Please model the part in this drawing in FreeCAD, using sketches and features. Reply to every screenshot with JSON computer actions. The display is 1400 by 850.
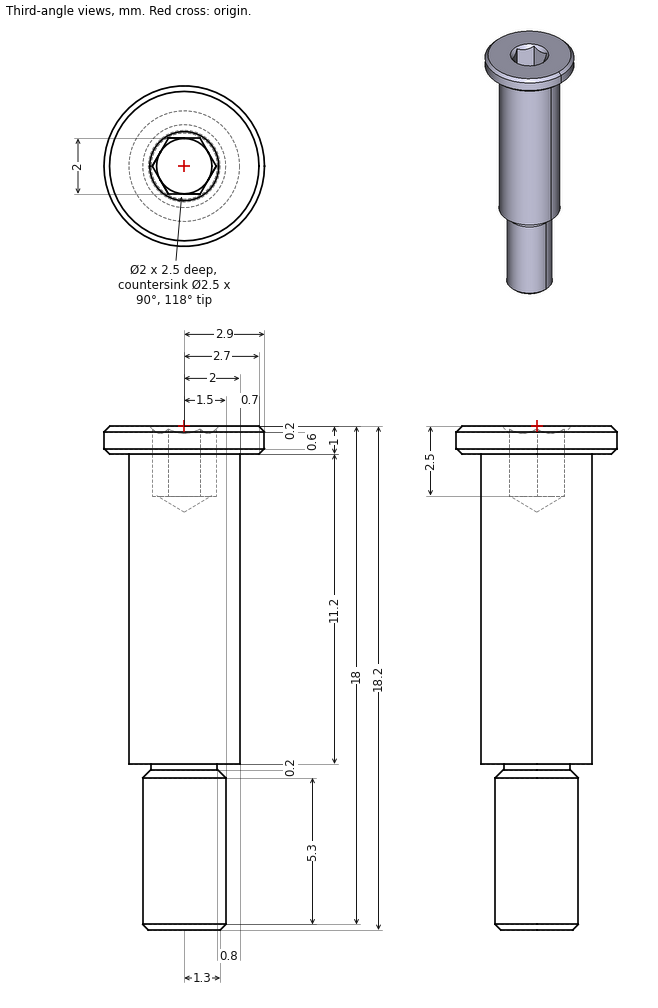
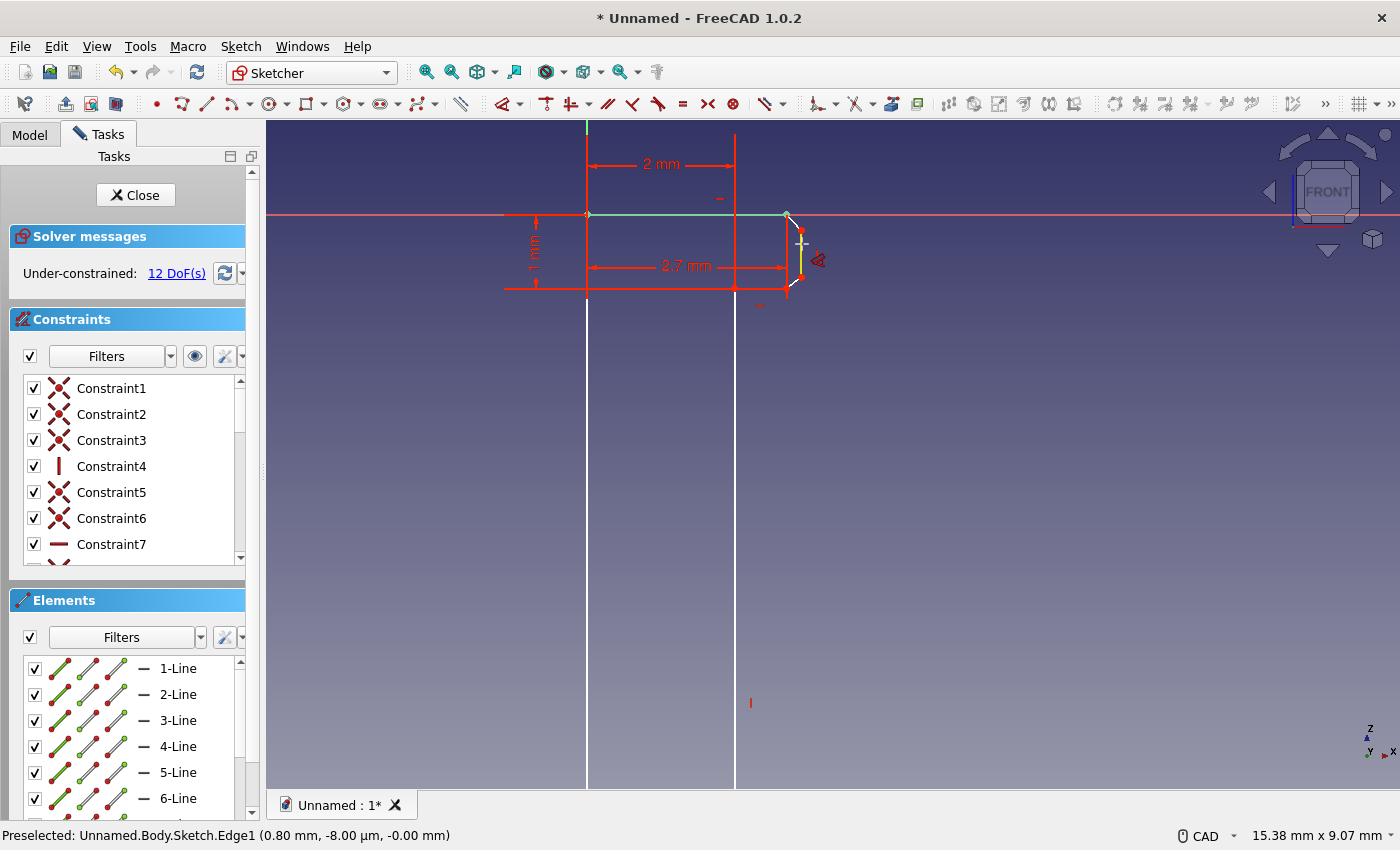
{"action": "left_click", "coordinate": [801, 244]}
{"action": "left_click", "coordinate": [835, 254]}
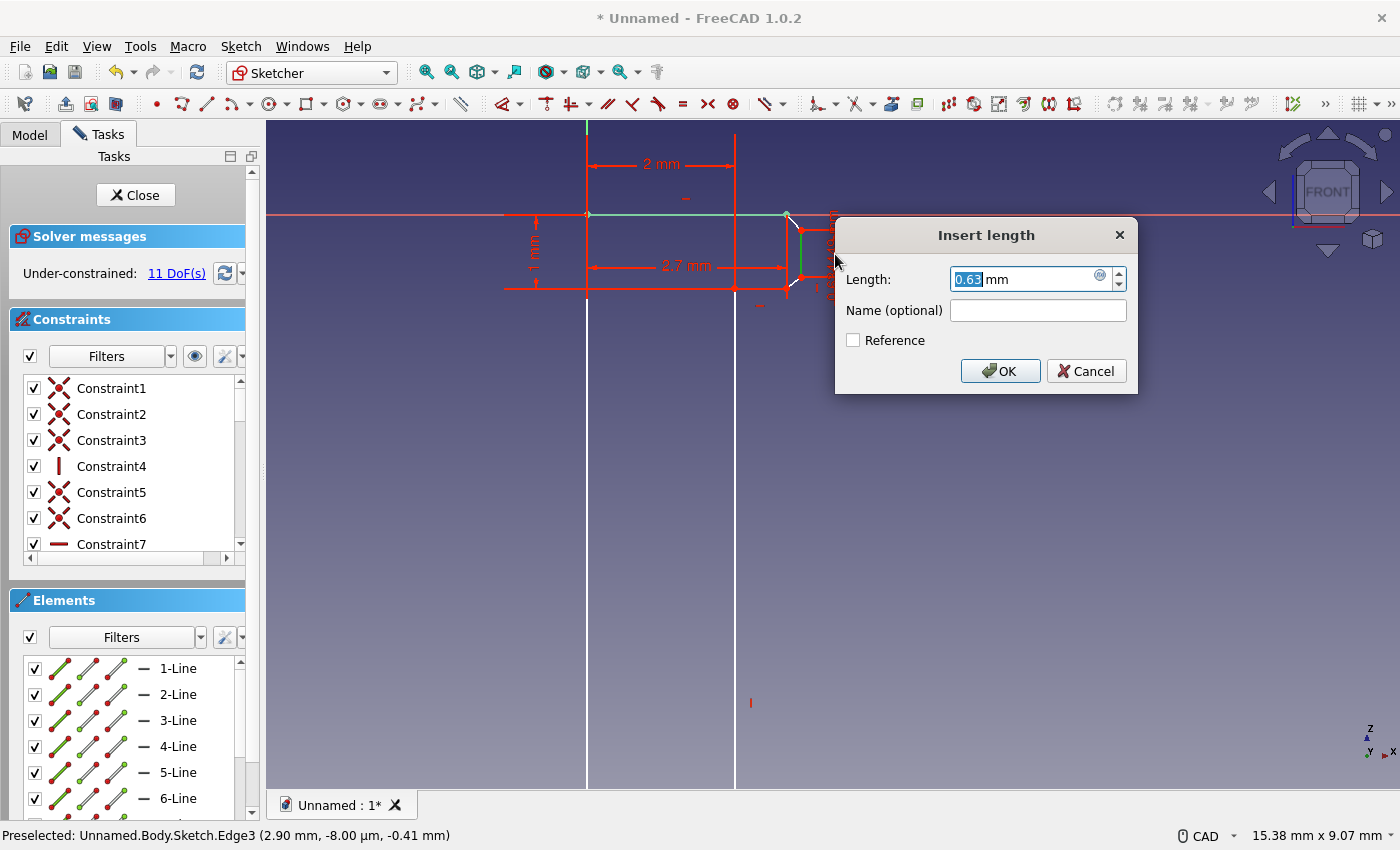
{"action": "type", "text": "0.6"}
{"action": "key", "text": "Return"}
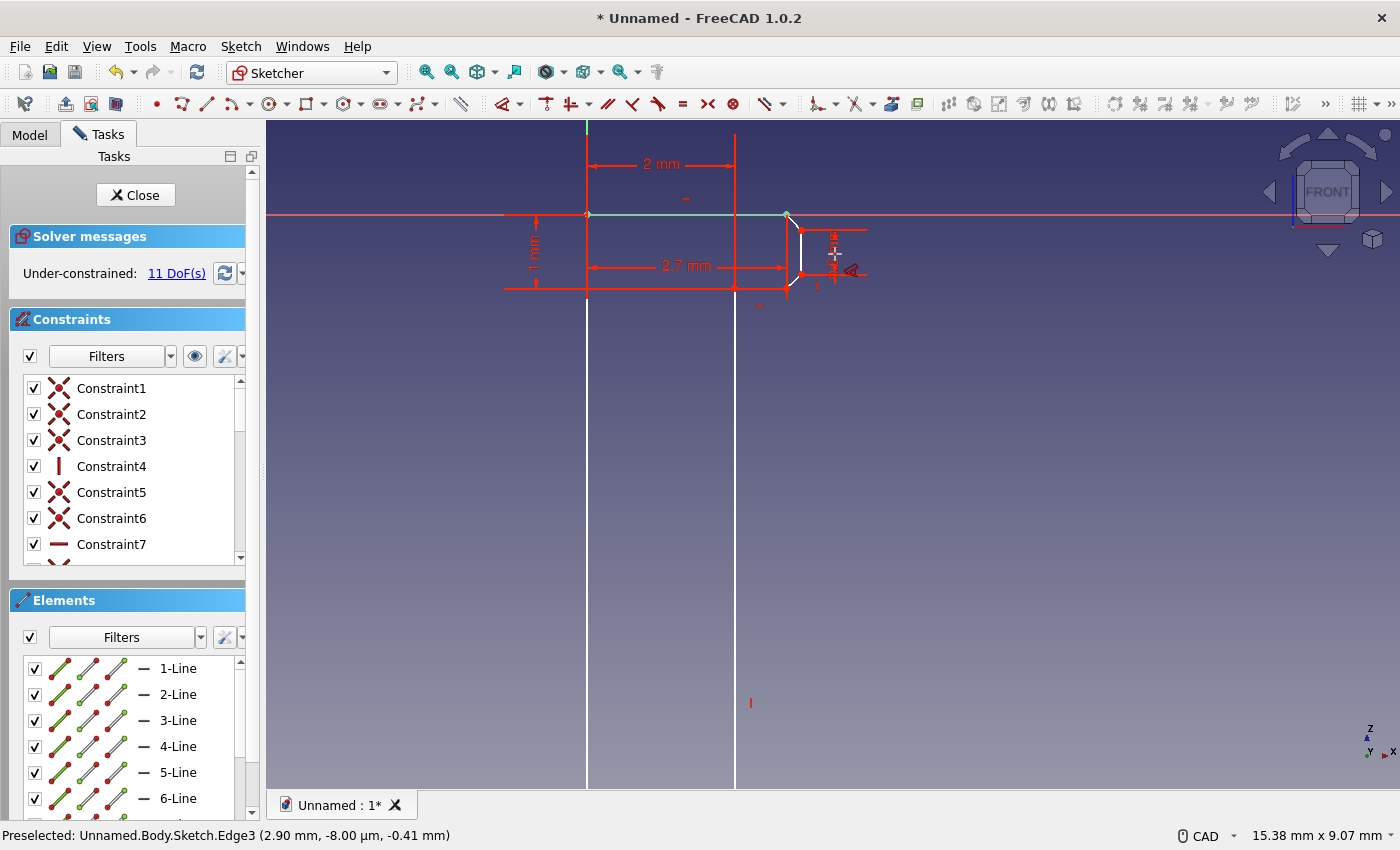
{"action": "left_click", "coordinate": [771, 289]}
{"action": "left_click", "coordinate": [760, 255]}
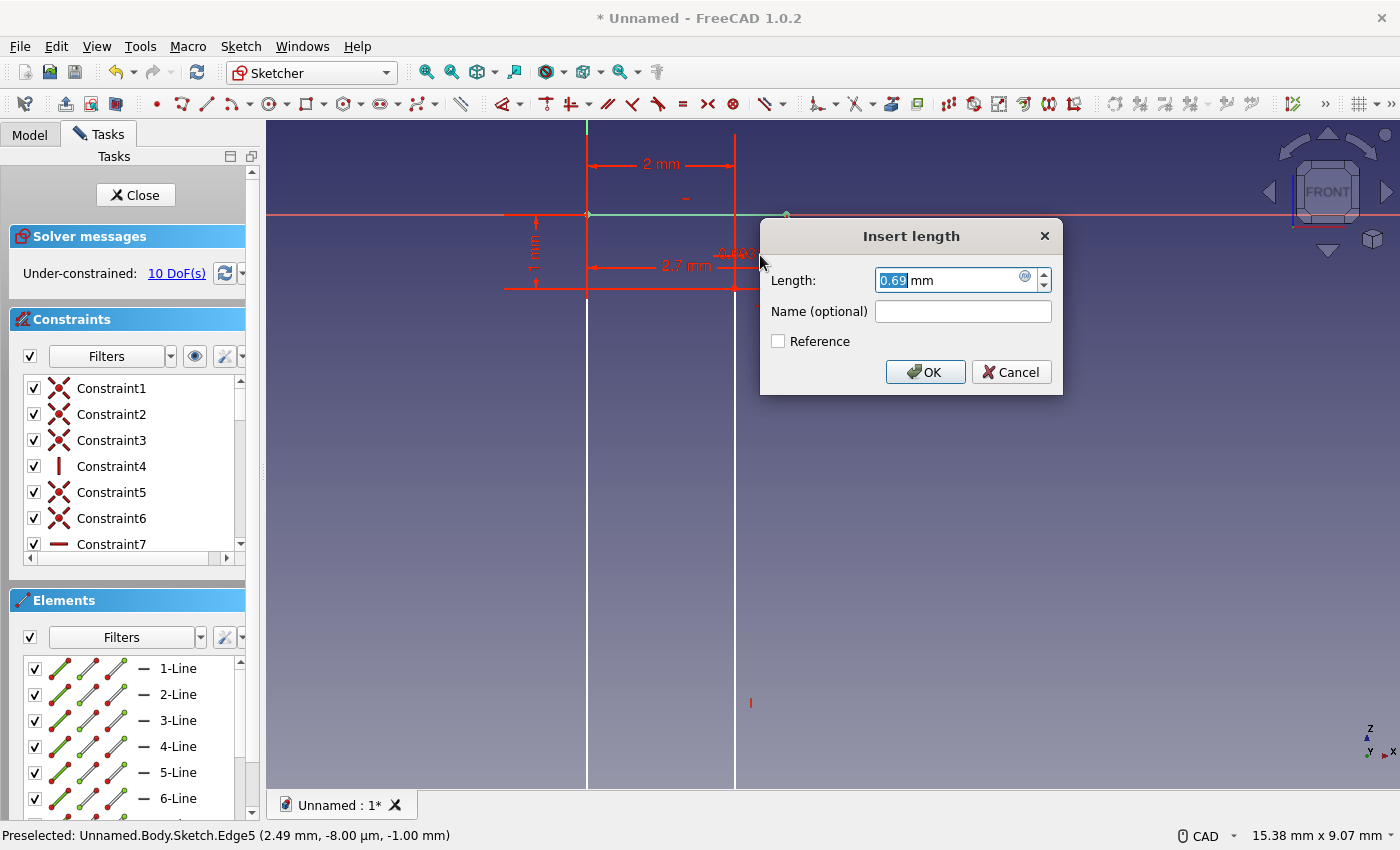
{"action": "type", "text": "0.7"}
{"action": "key", "text": "Return"}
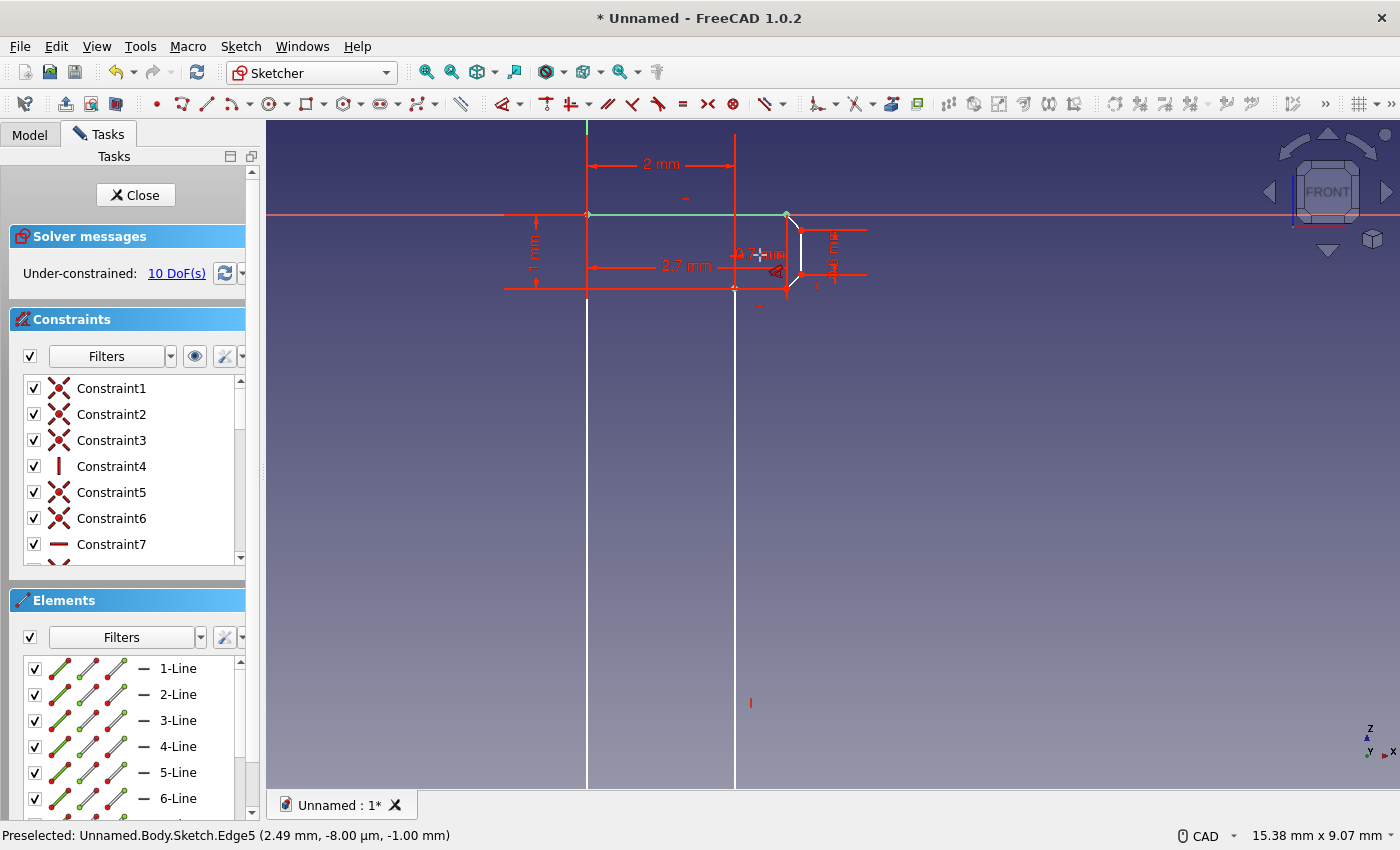
{"action": "scroll", "coordinate": [795, 268], "scroll_direction": "down", "scroll_amount": 6}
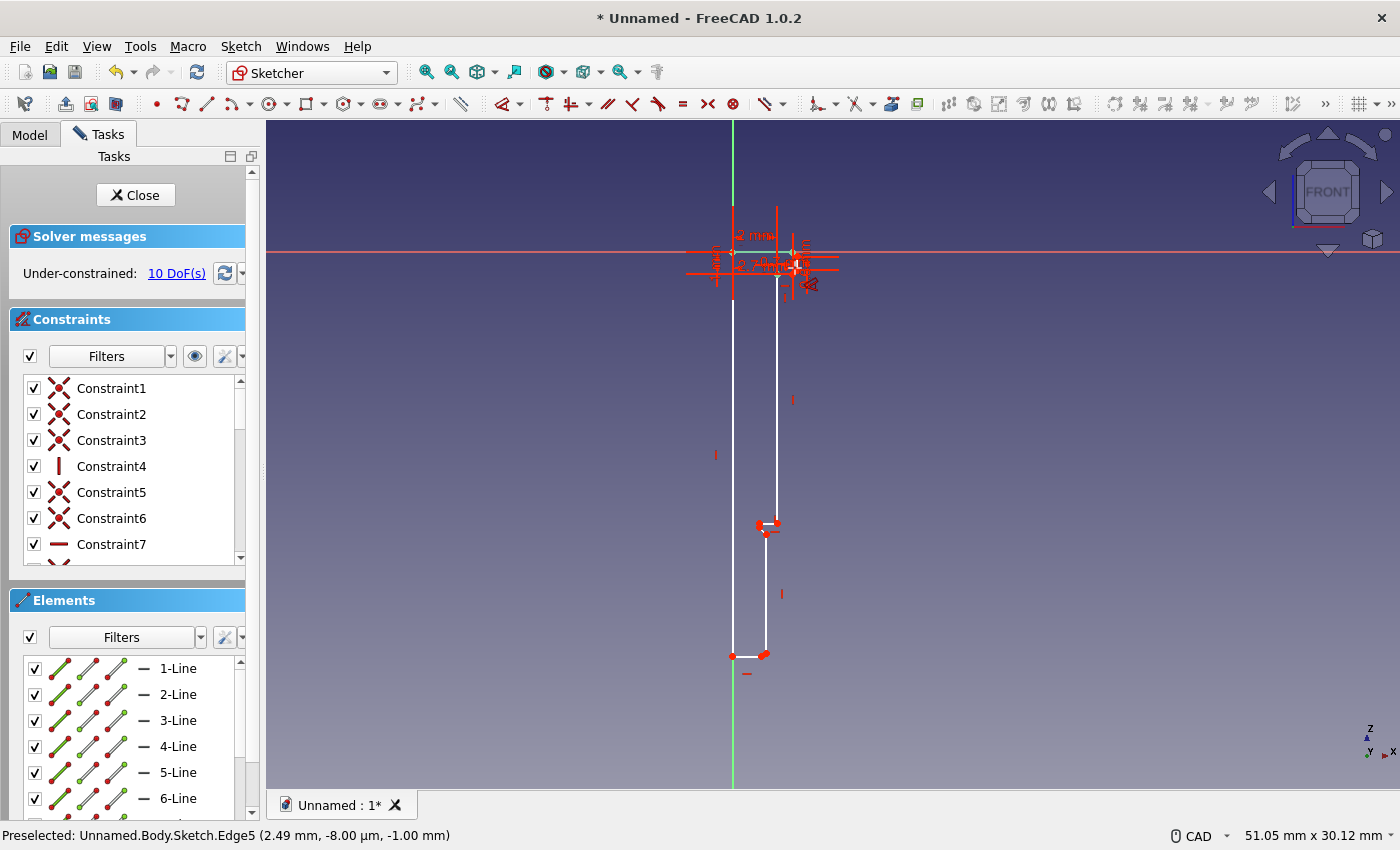
{"action": "scroll", "coordinate": [772, 524], "scroll_direction": "up", "scroll_amount": 5}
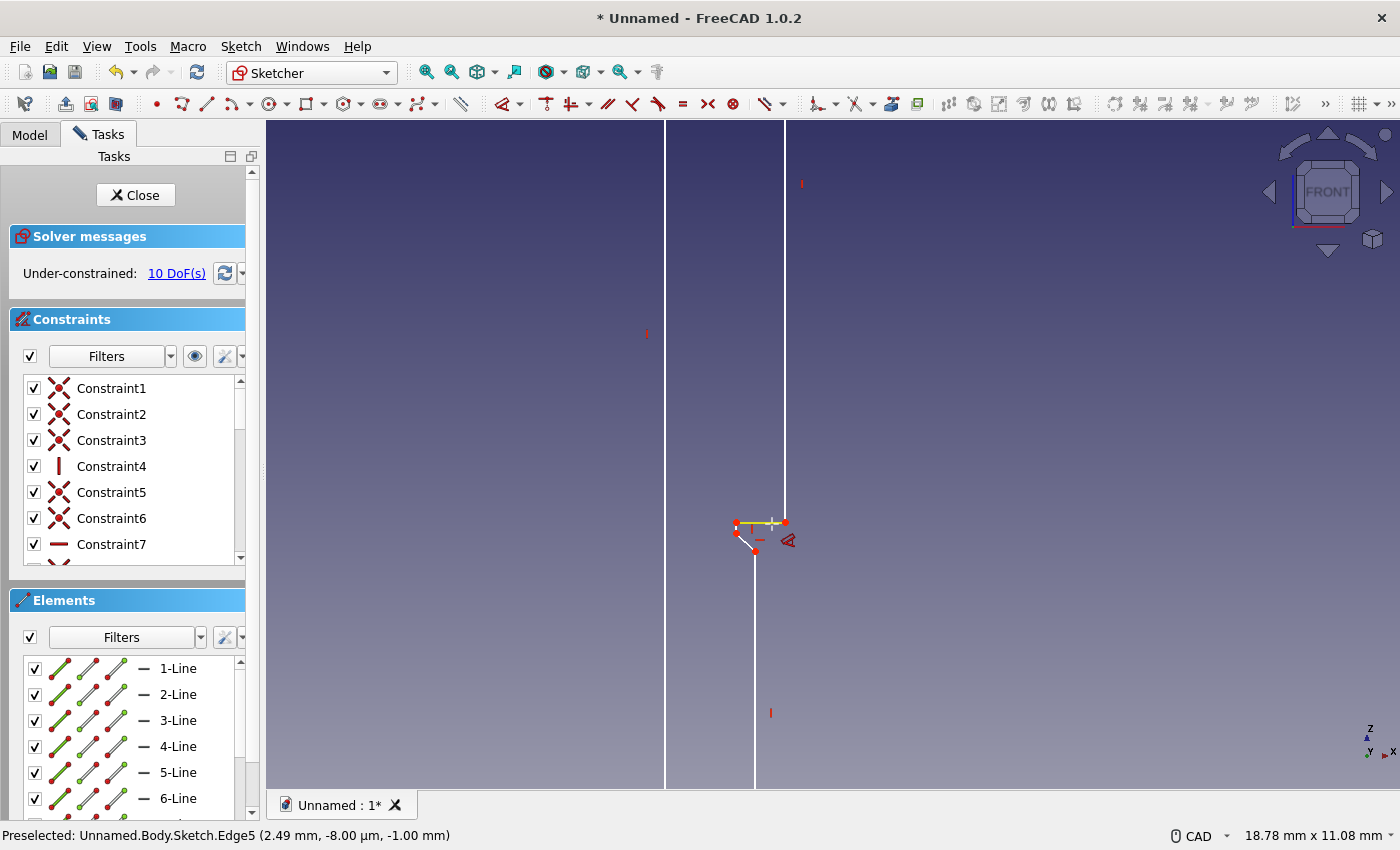
{"action": "left_click", "coordinate": [771, 523]}
{"action": "left_click", "coordinate": [772, 557]}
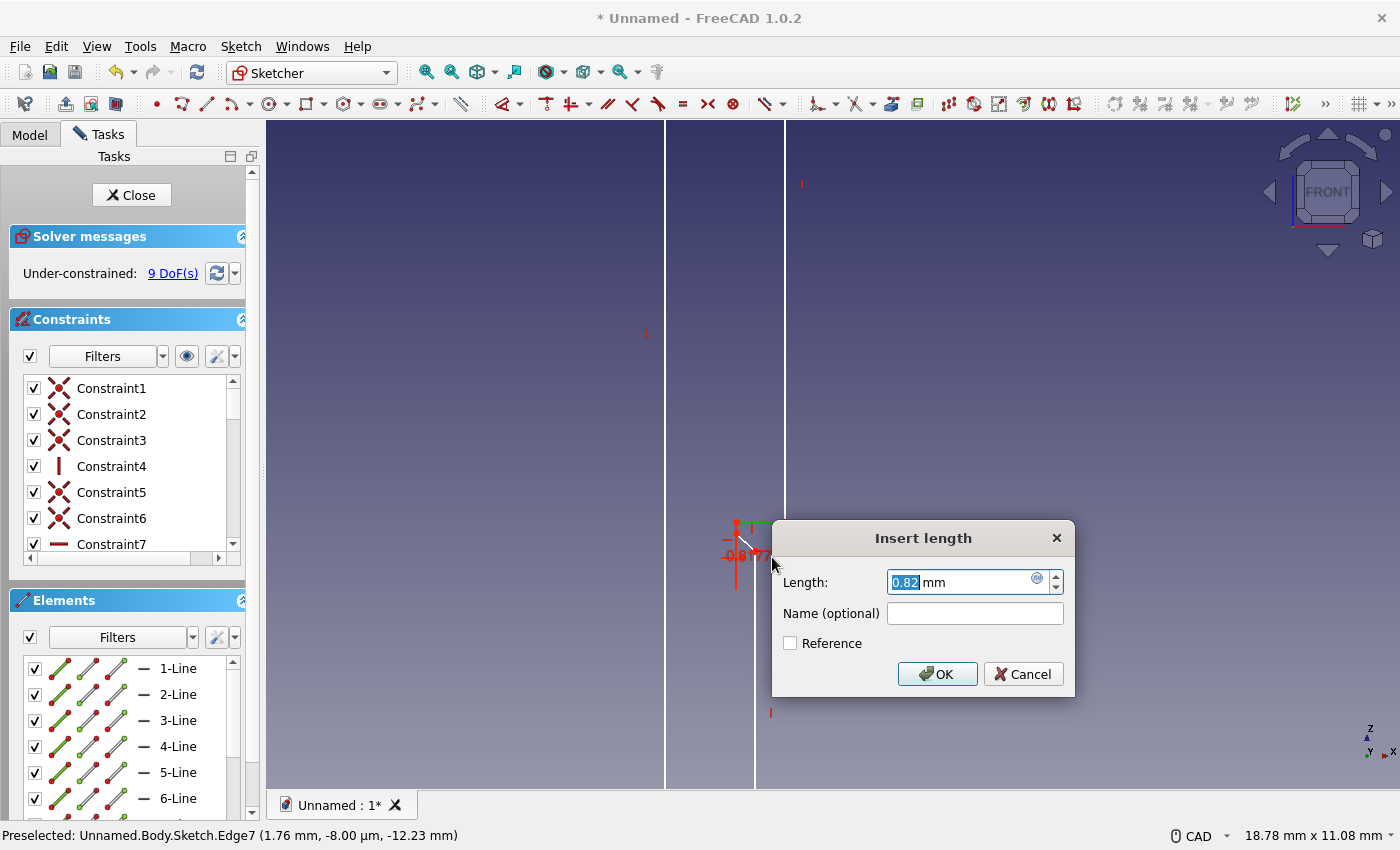
{"action": "type", "text": "0.8"}
{"action": "key", "text": "Return"}